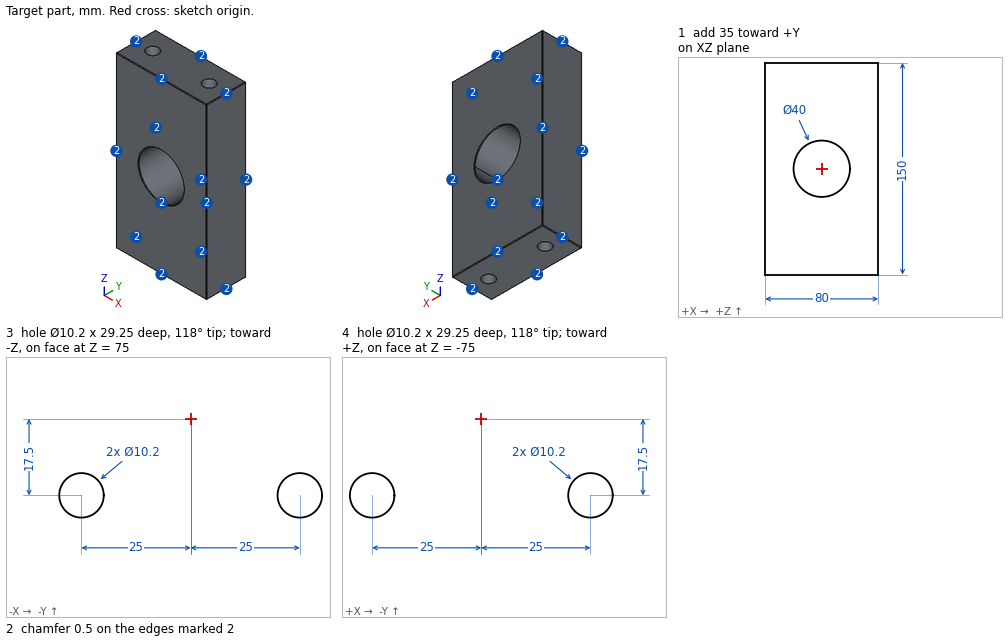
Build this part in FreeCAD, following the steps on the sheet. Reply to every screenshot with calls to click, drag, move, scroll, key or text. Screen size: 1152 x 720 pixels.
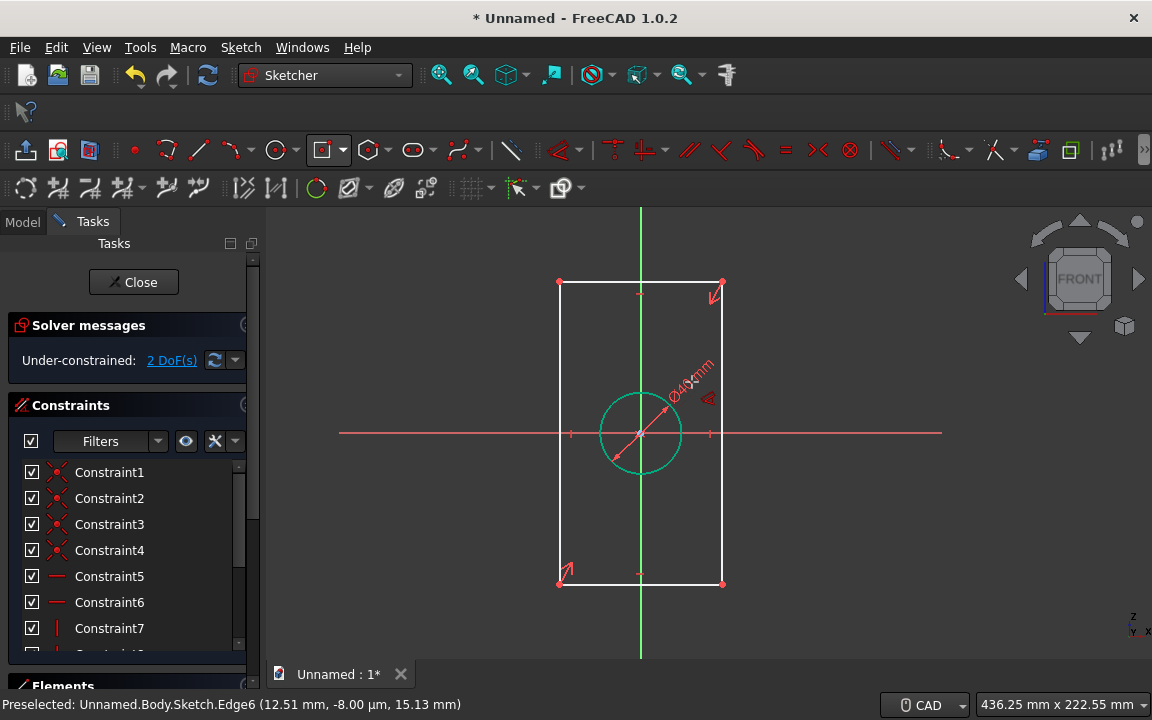
click(608, 585)
click(604, 619)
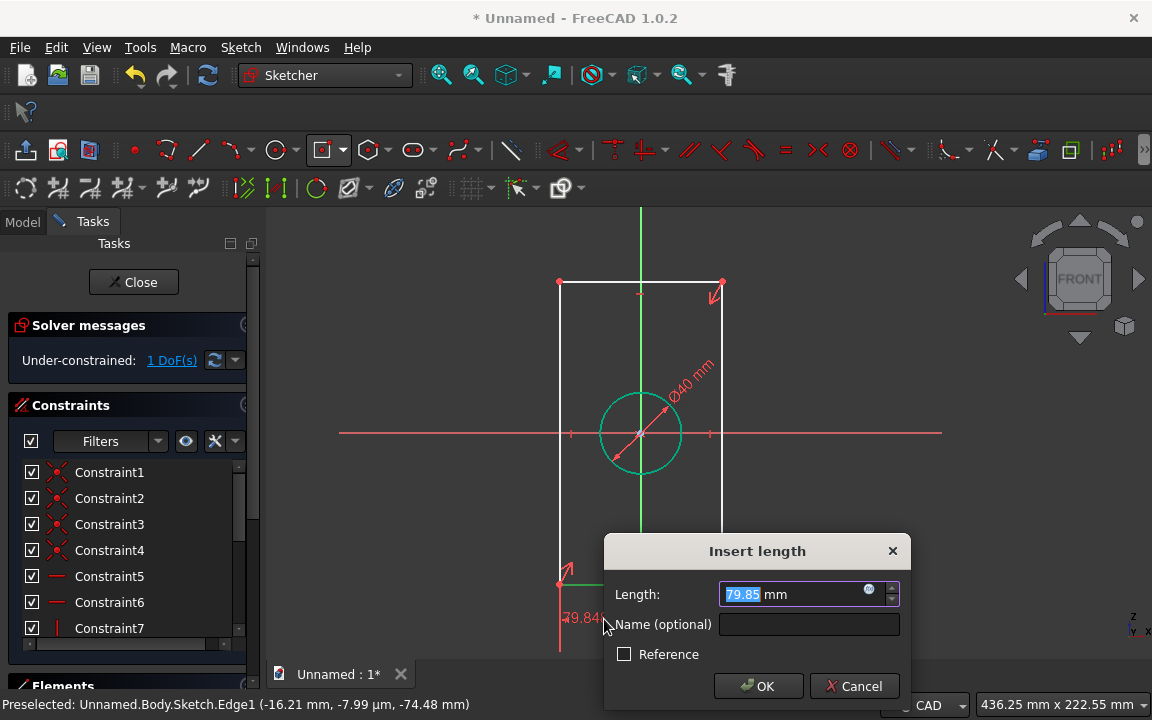
text(80)
key(Return)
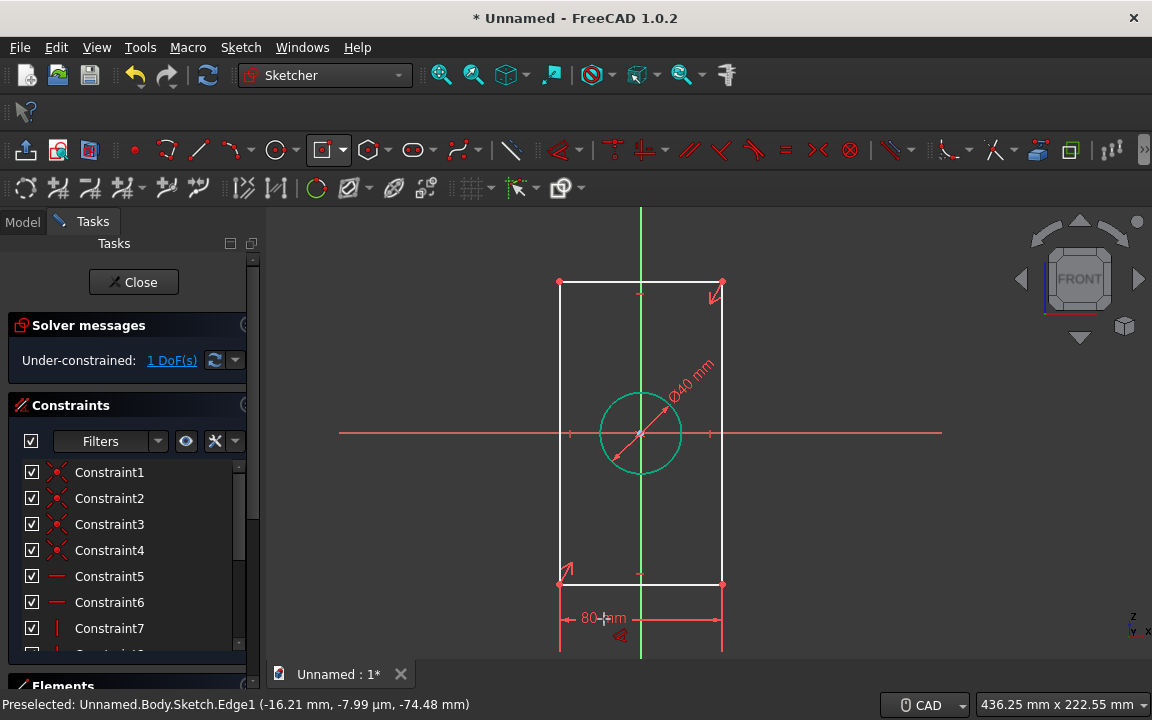
click(722, 494)
click(756, 503)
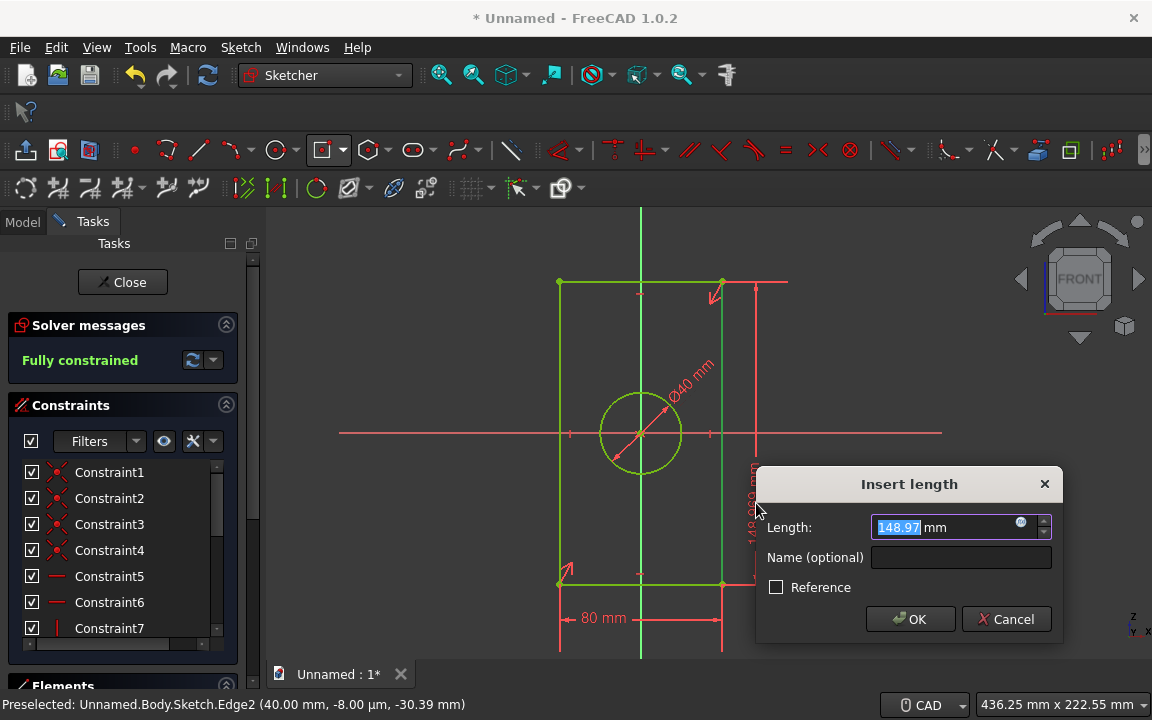
text(150)
key(Return)
key(Escape)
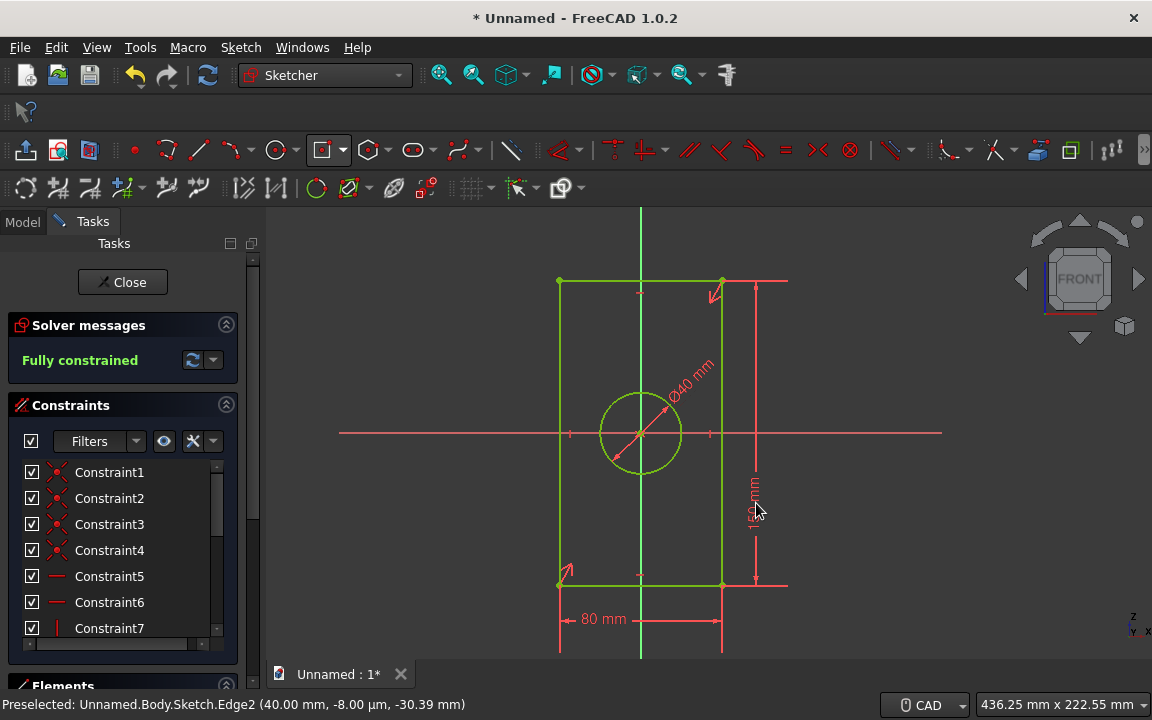
click(123, 282)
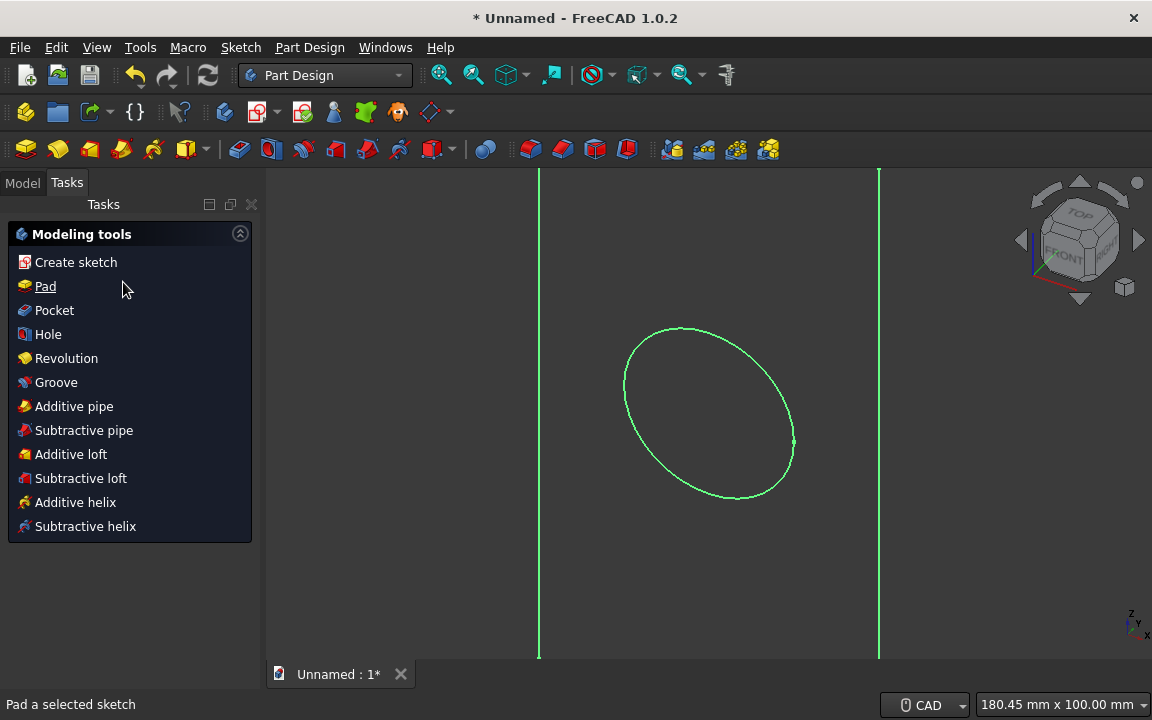
click(26, 150)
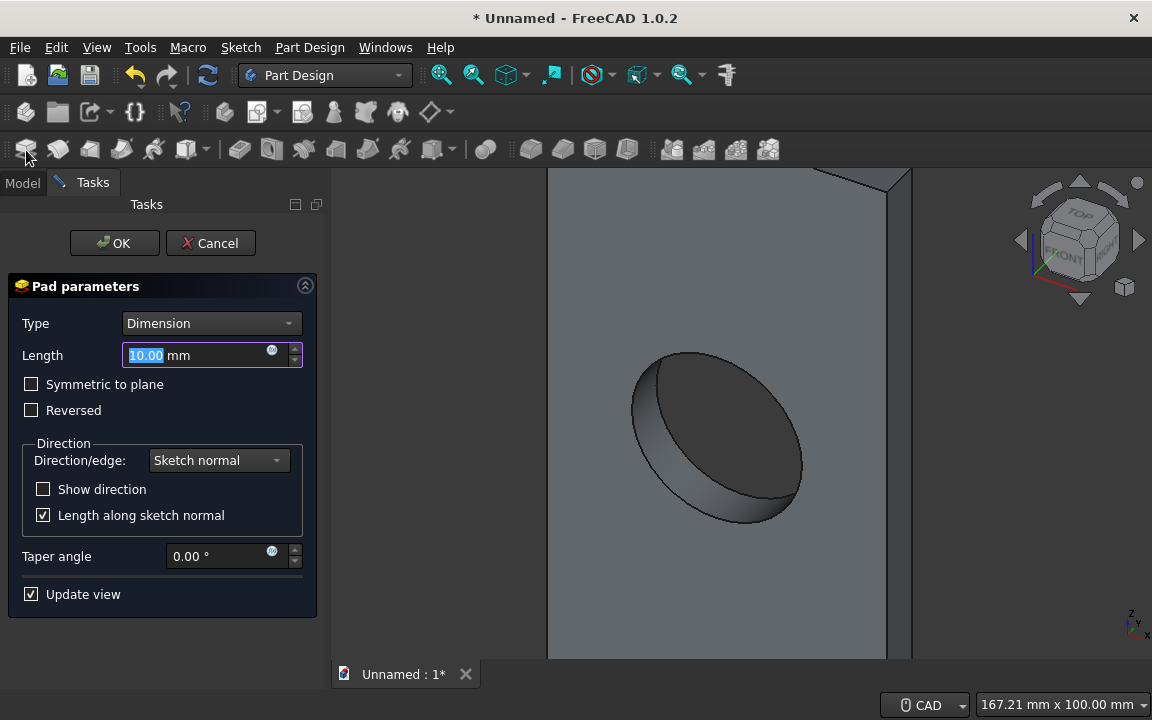
text(35)
key(Tab)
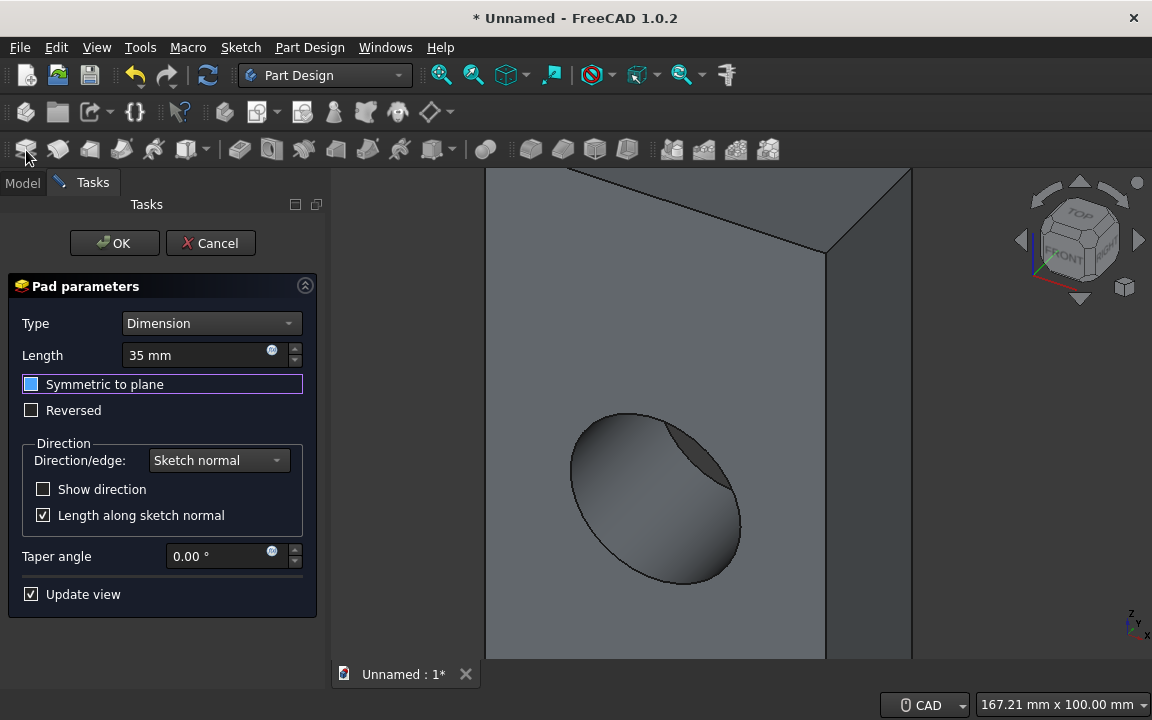
click(30, 410)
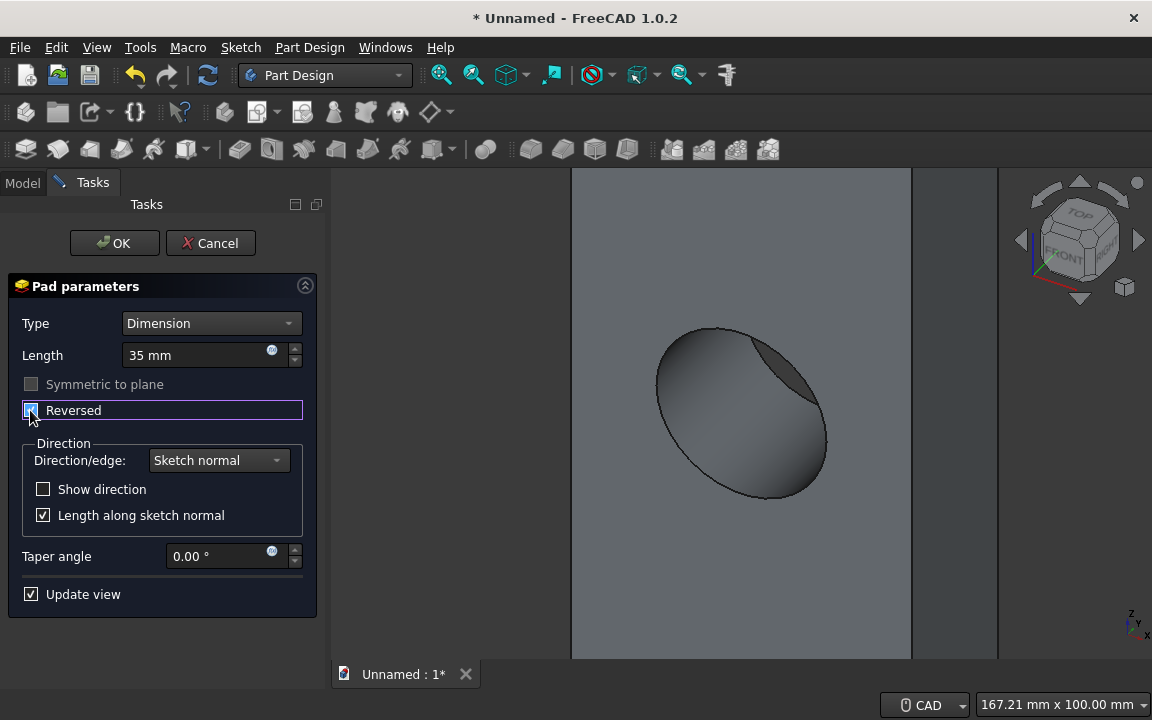
click(115, 243)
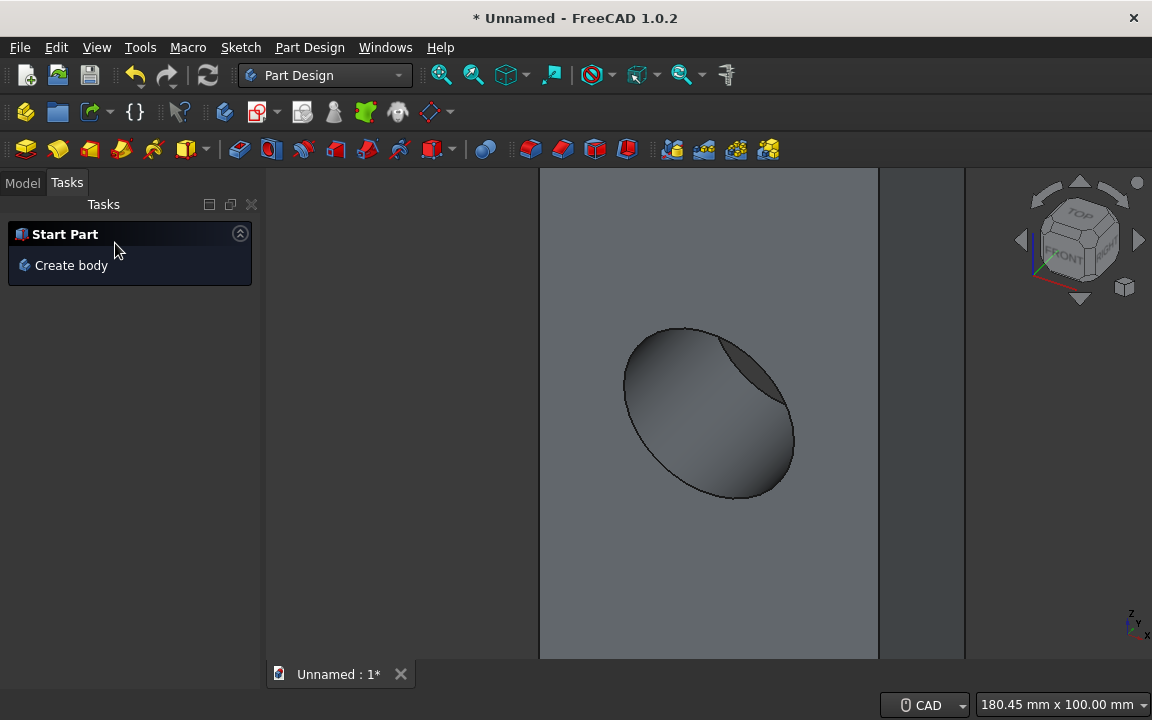
click(442, 76)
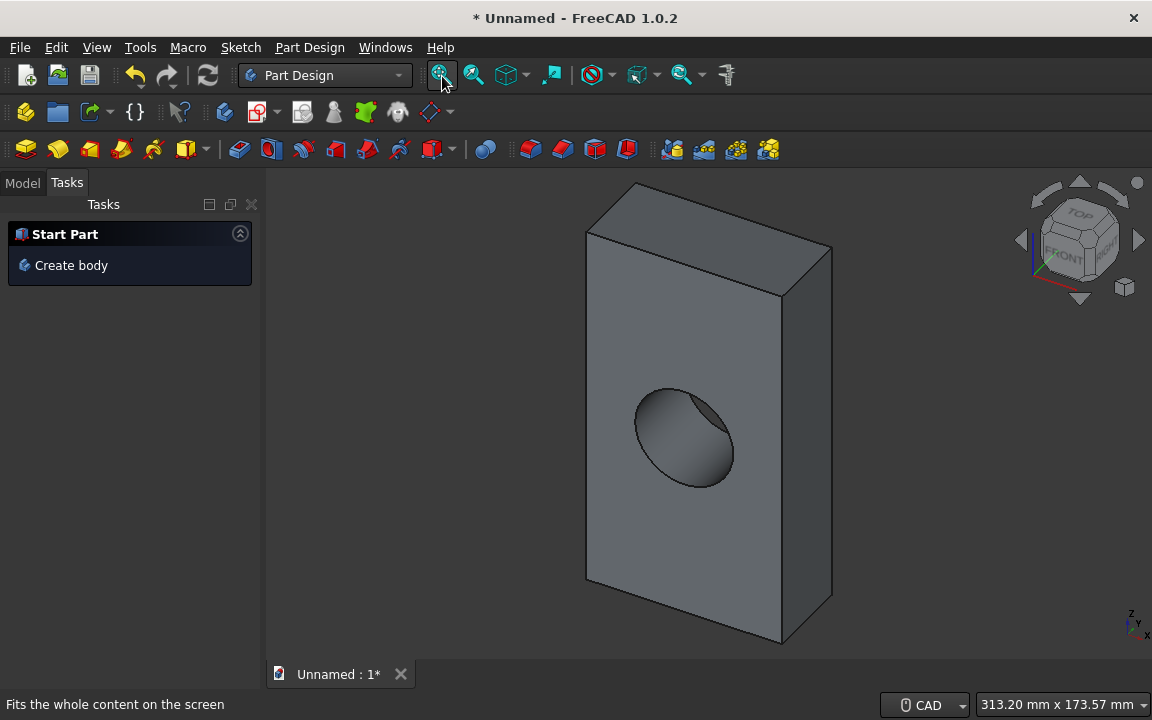
click(712, 347)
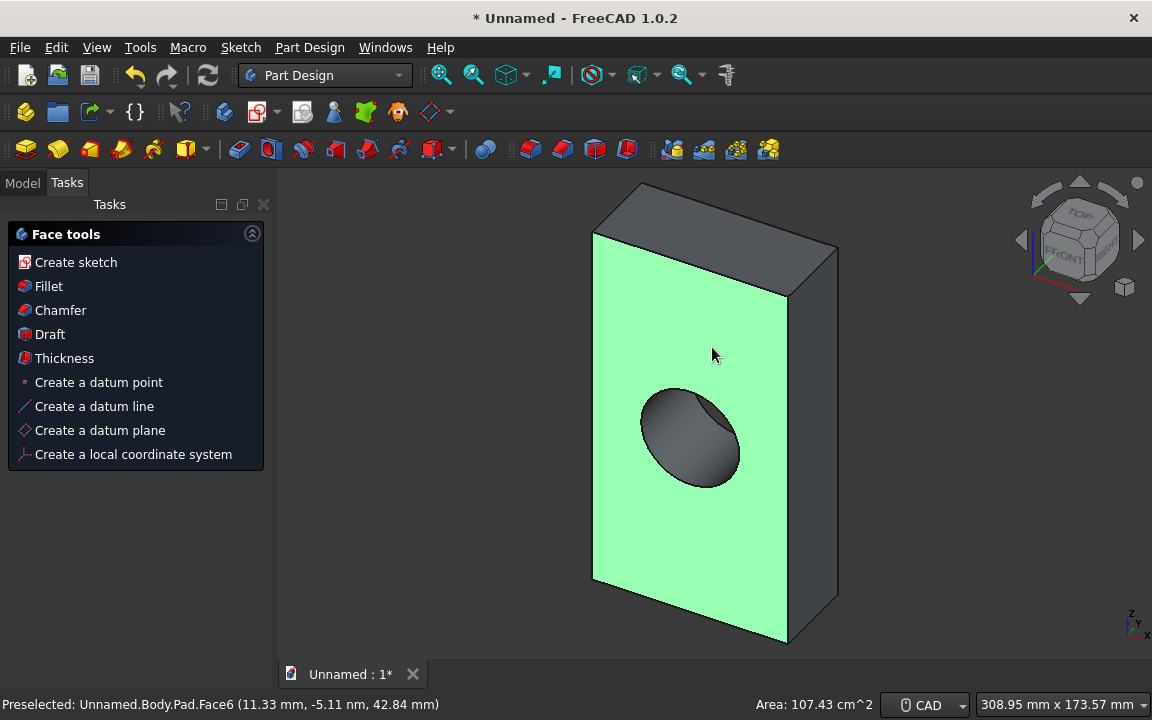
click(813, 271, ctrl)